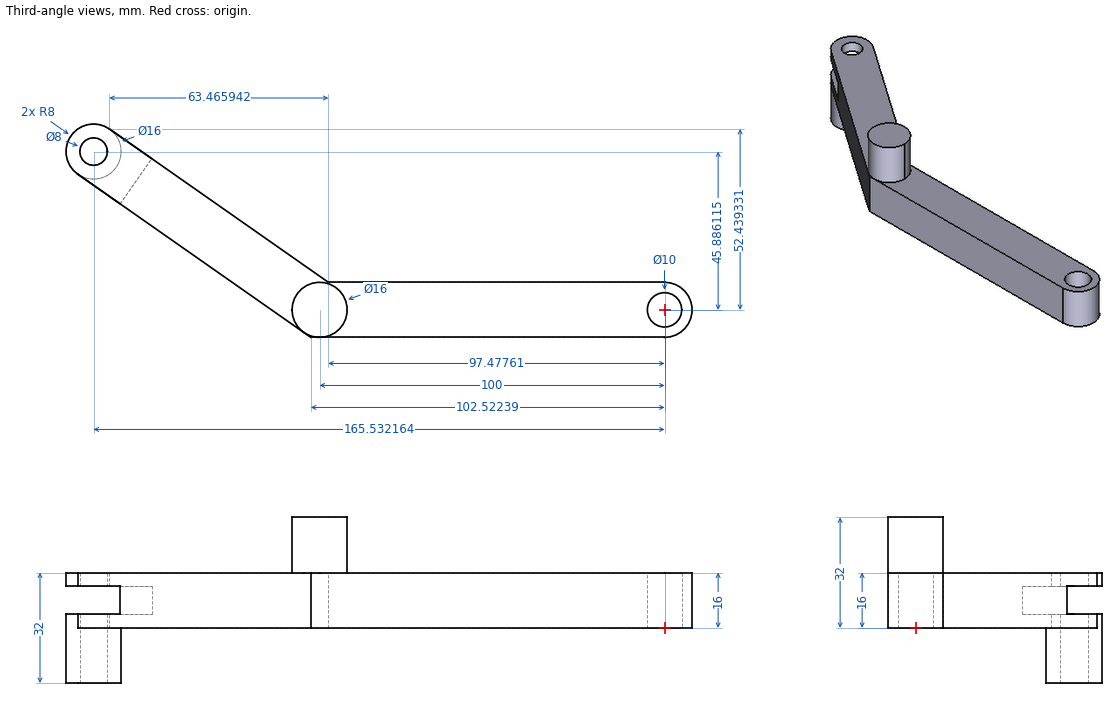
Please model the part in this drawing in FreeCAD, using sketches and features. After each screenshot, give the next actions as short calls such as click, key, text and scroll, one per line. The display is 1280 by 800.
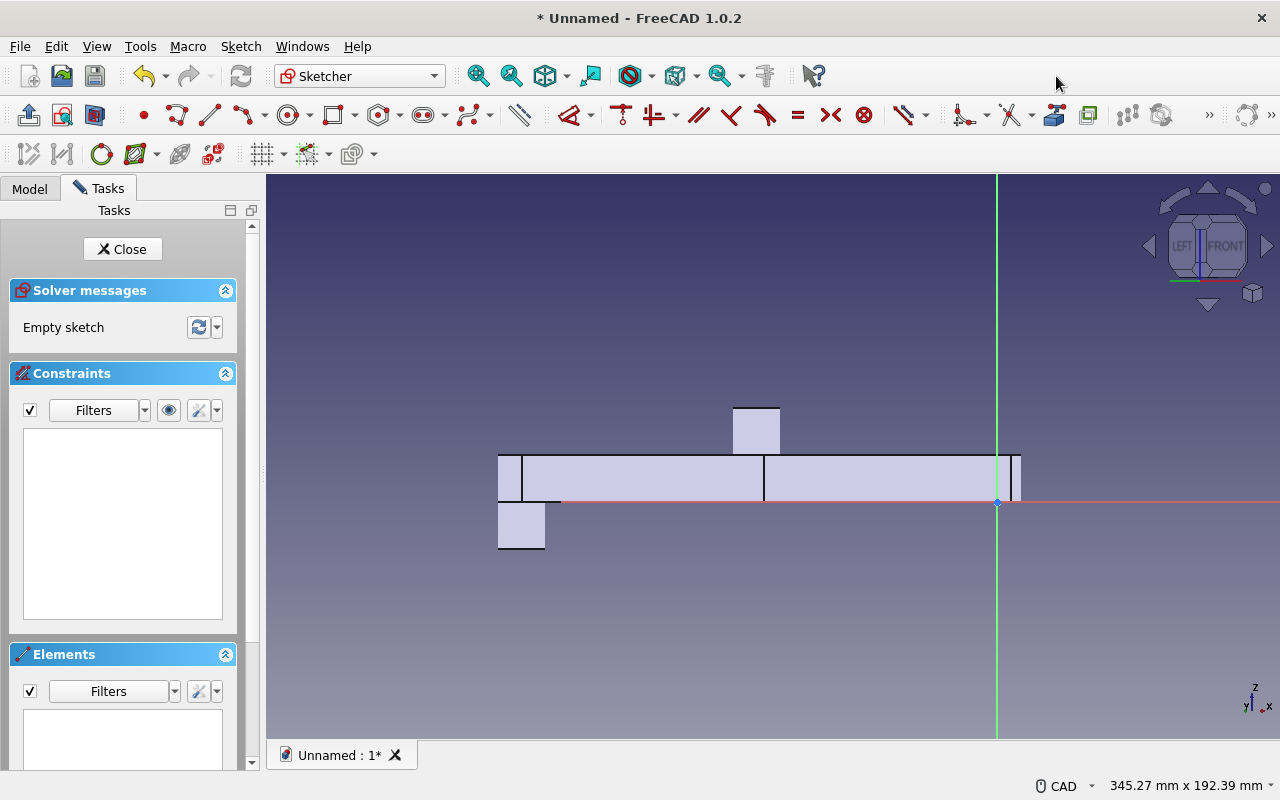
scroll(486, 483, up, 9)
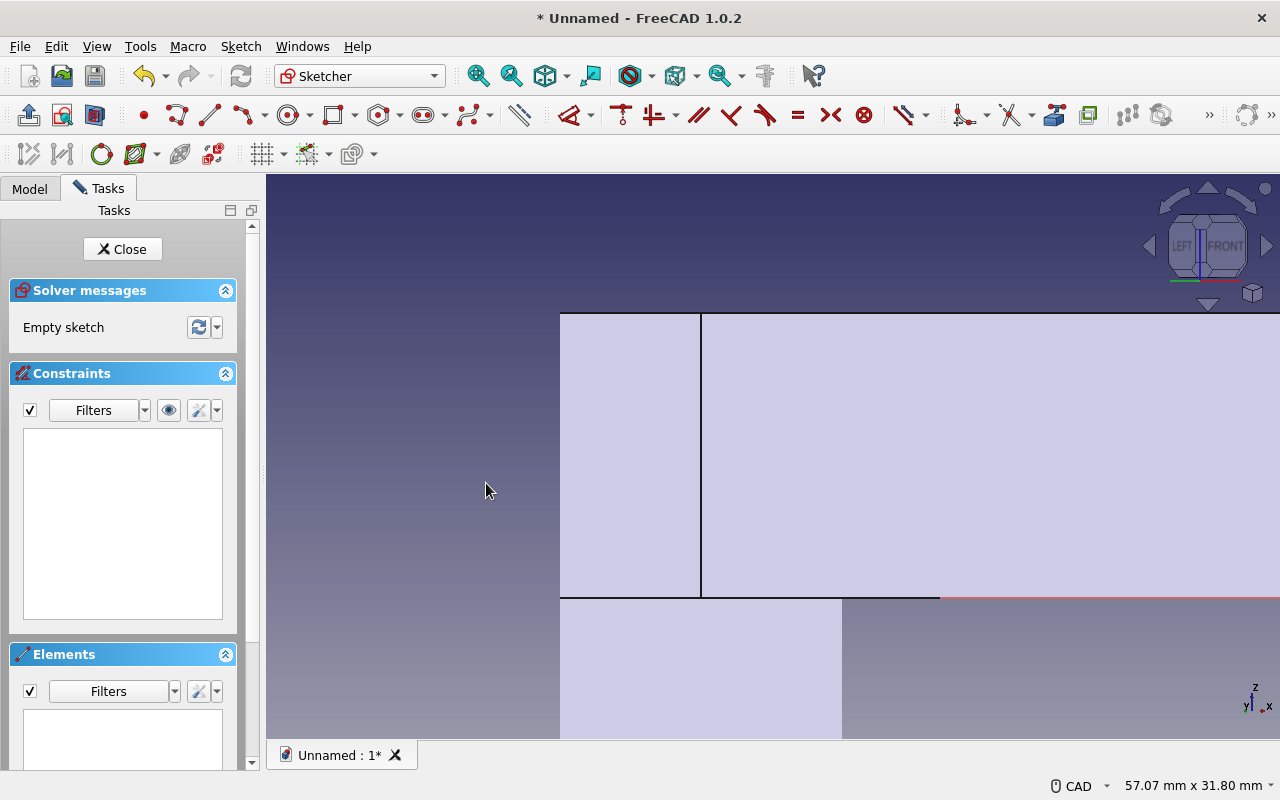
click(332, 116)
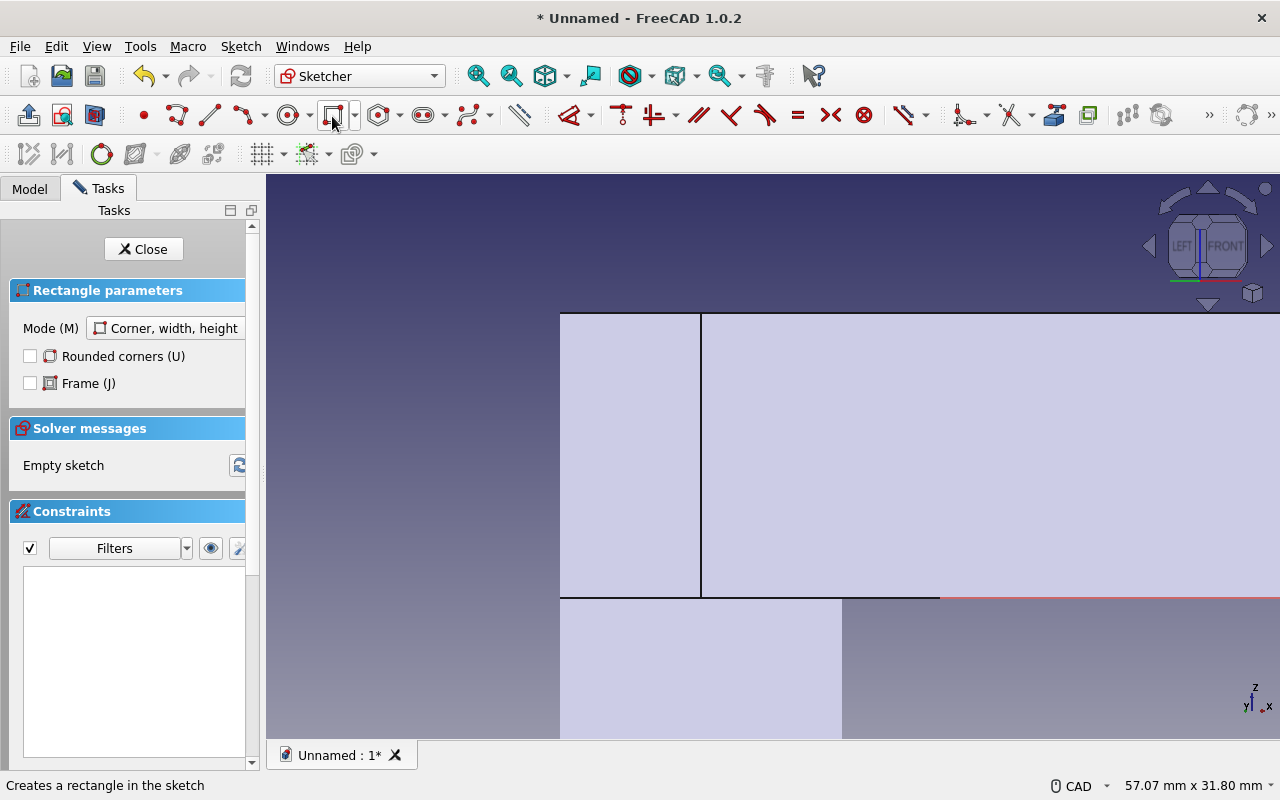
click(435, 384)
click(968, 526)
key(Escape)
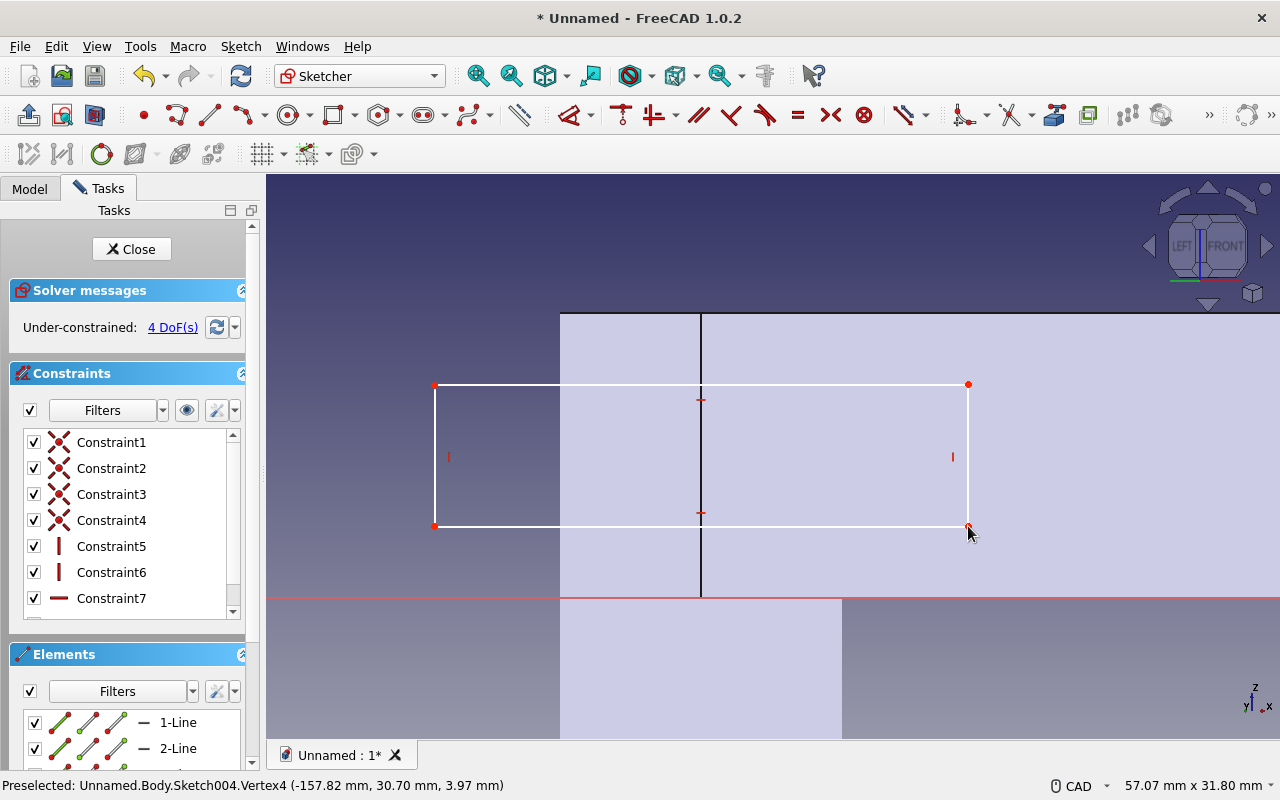
key(d)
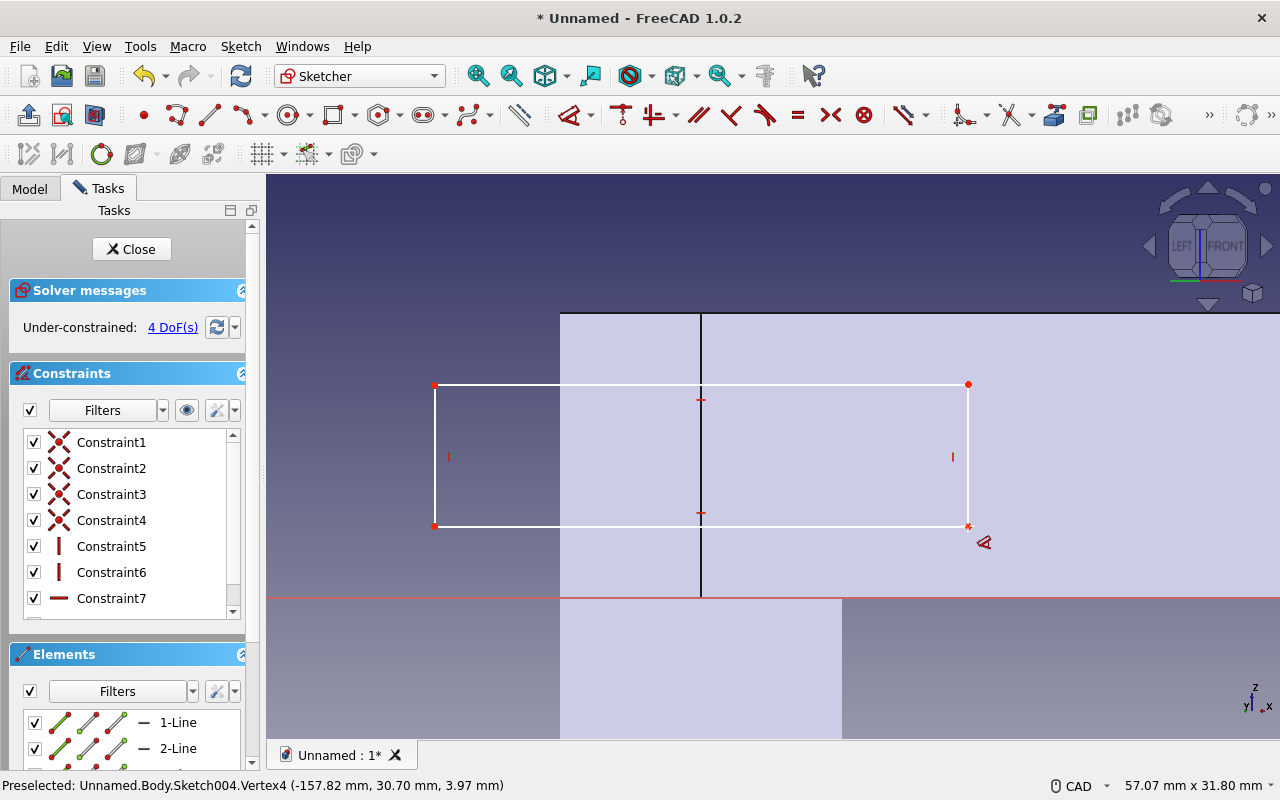
click(435, 428)
click(401, 456)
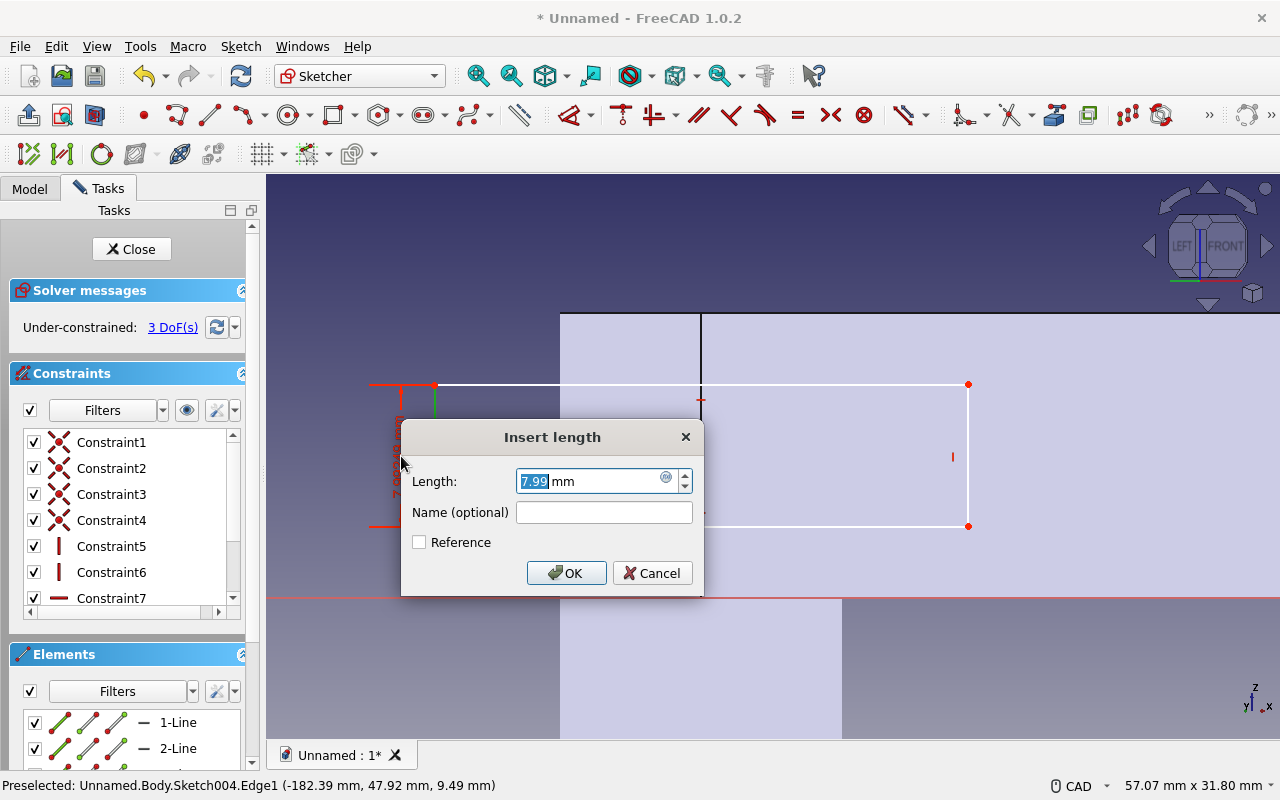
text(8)
key(Return)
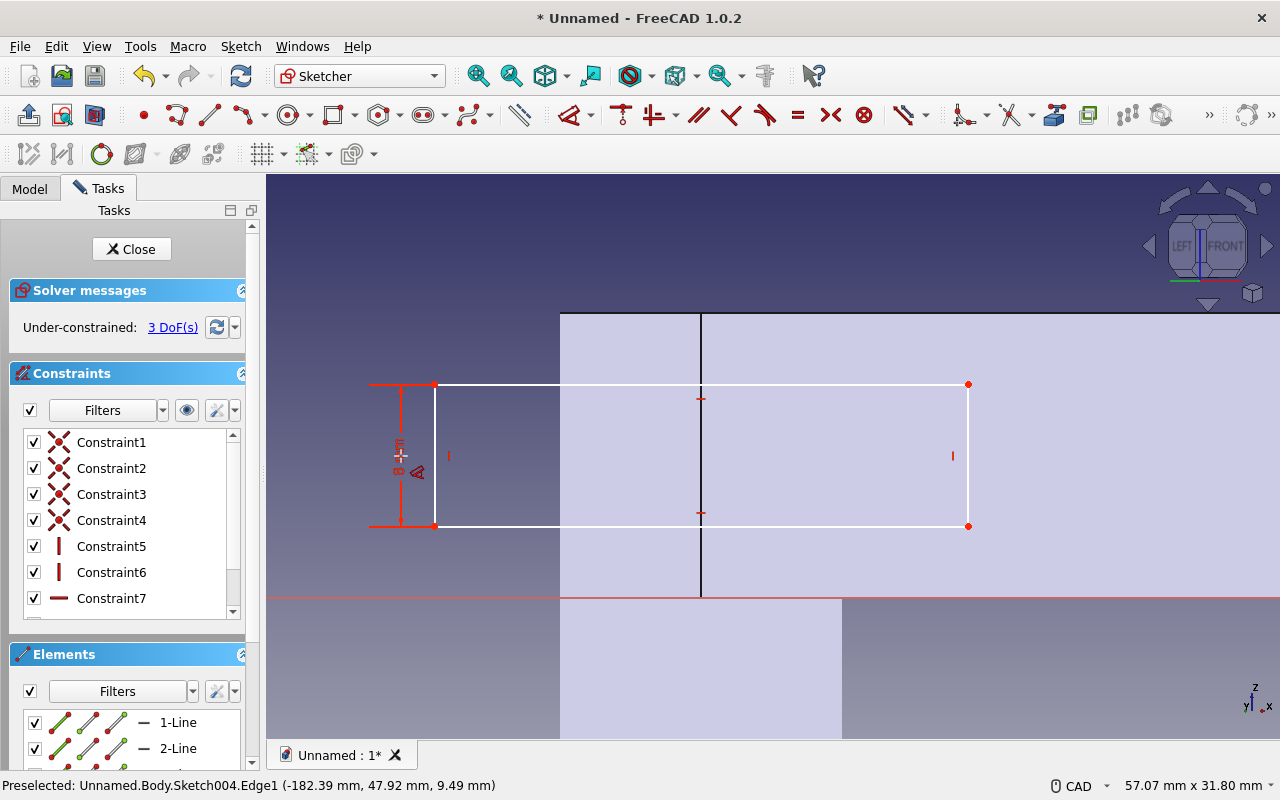
click(595, 527)
click(702, 561)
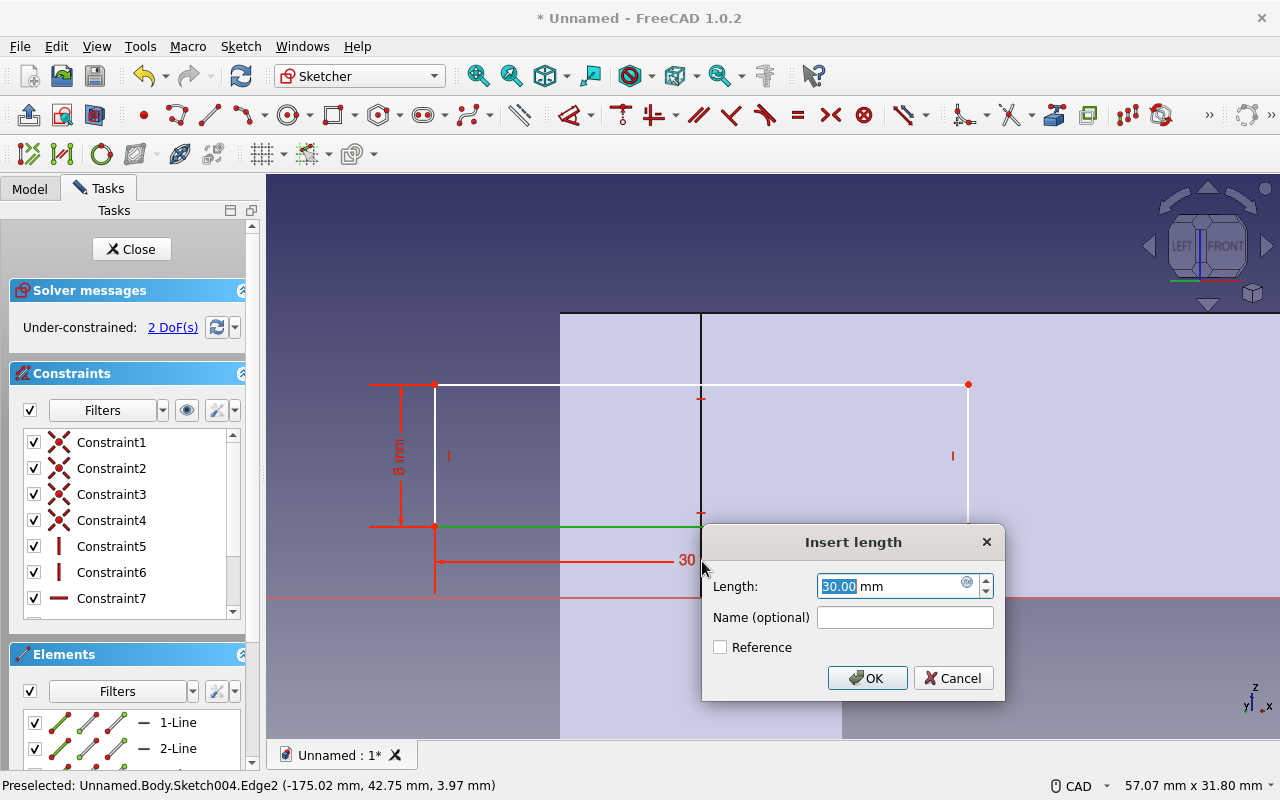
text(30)
key(Return)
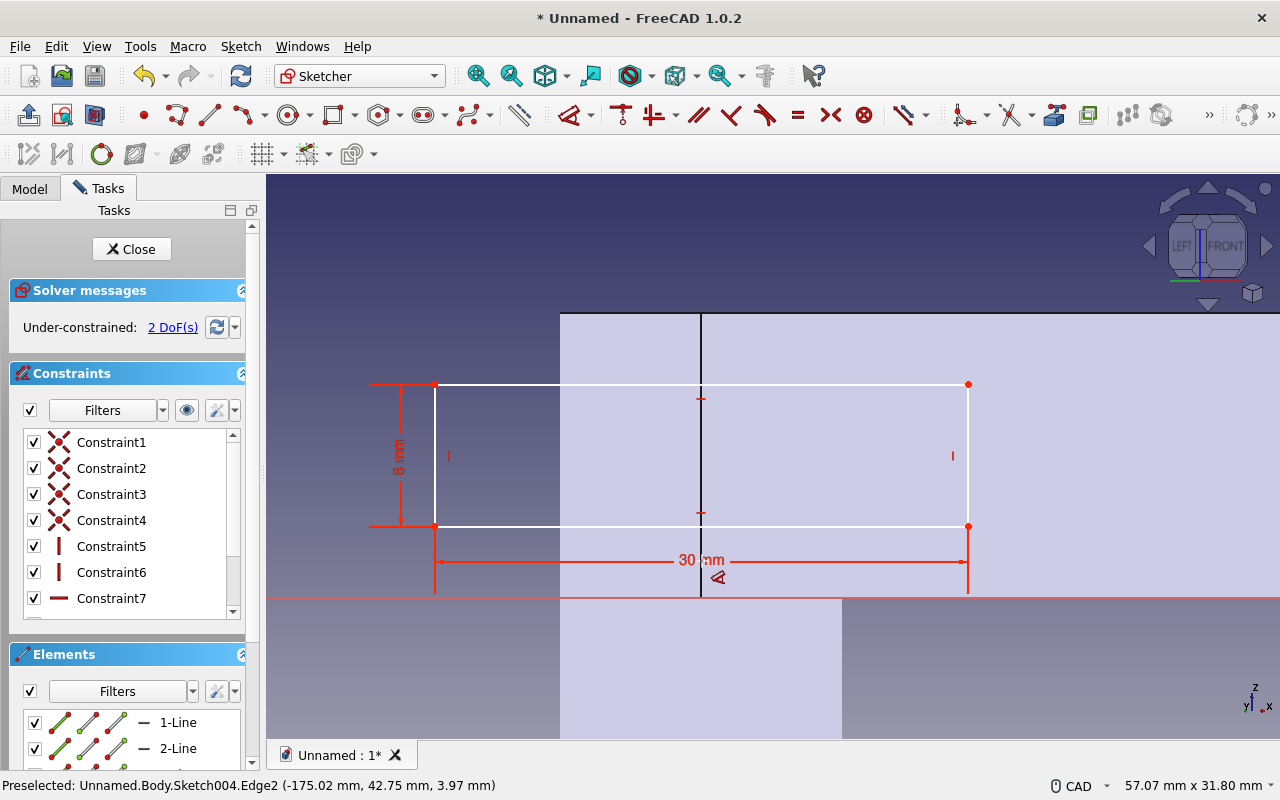
click(435, 527)
click(401, 562)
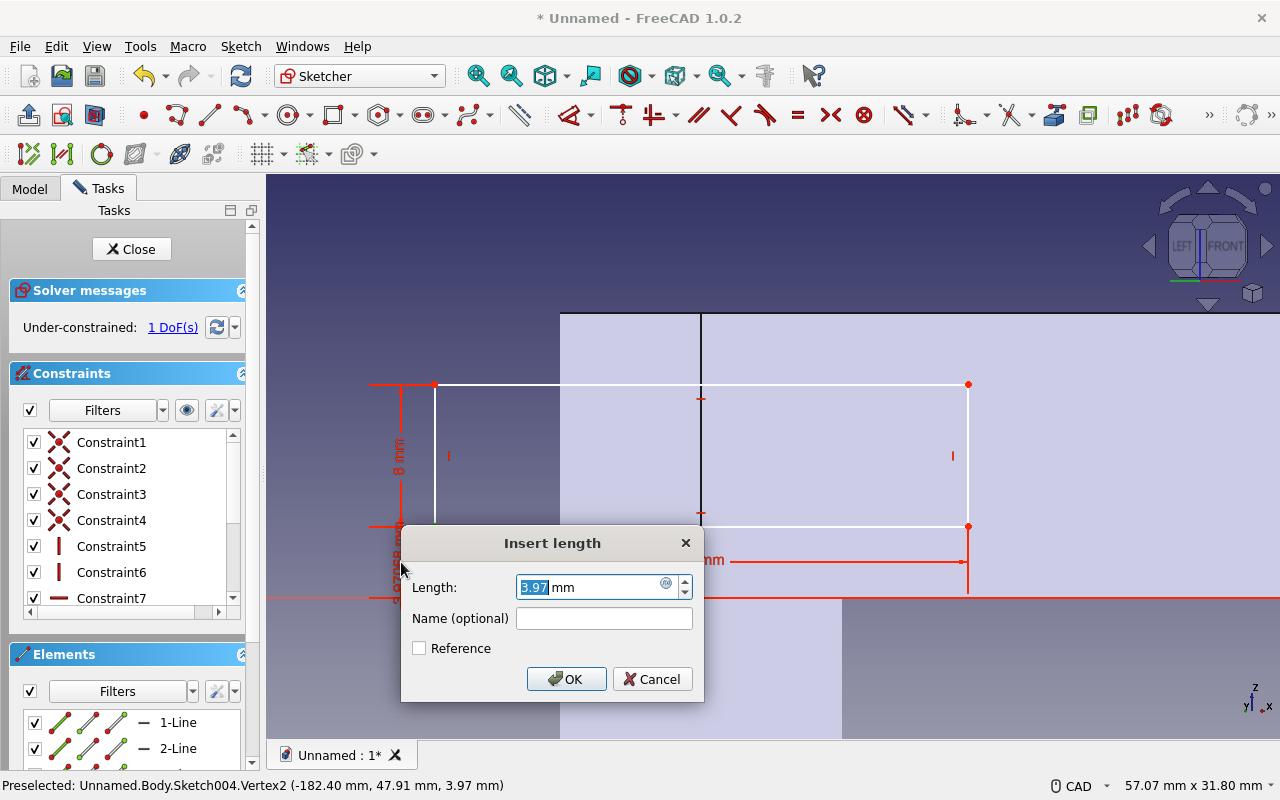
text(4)
key(Return)